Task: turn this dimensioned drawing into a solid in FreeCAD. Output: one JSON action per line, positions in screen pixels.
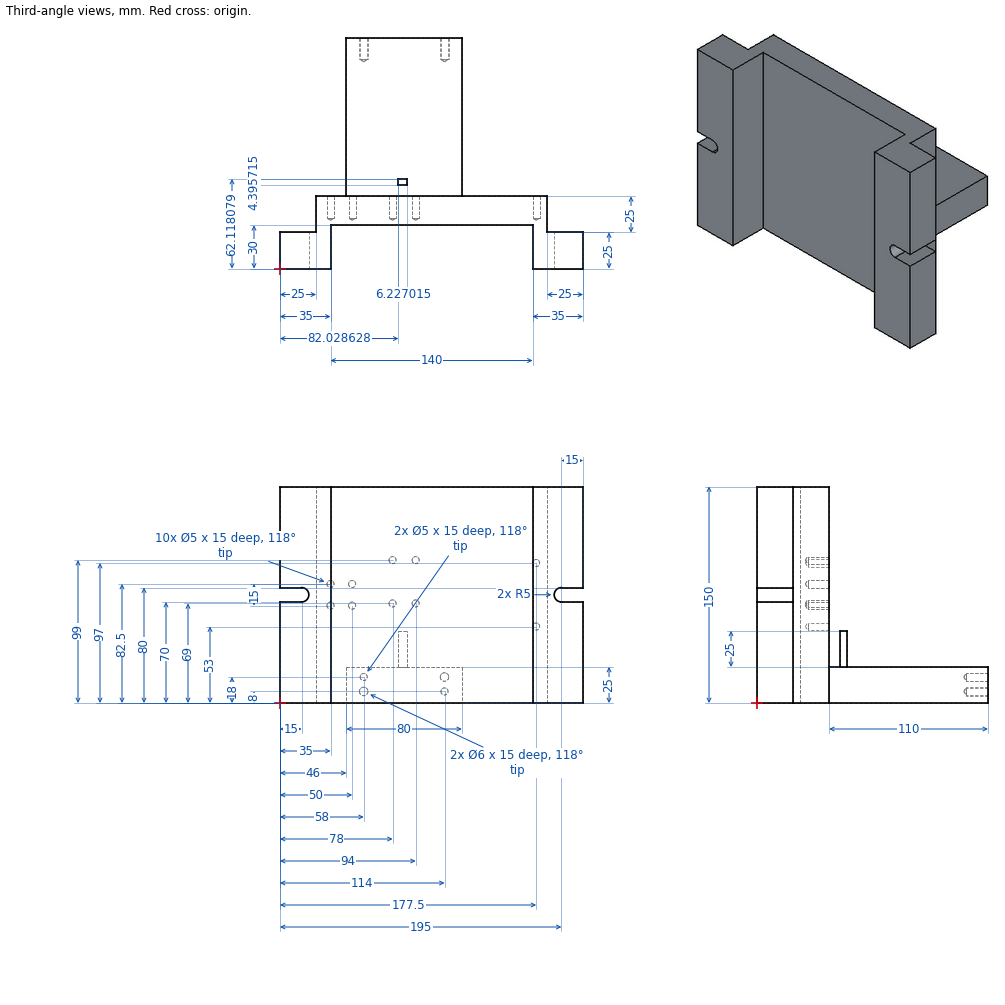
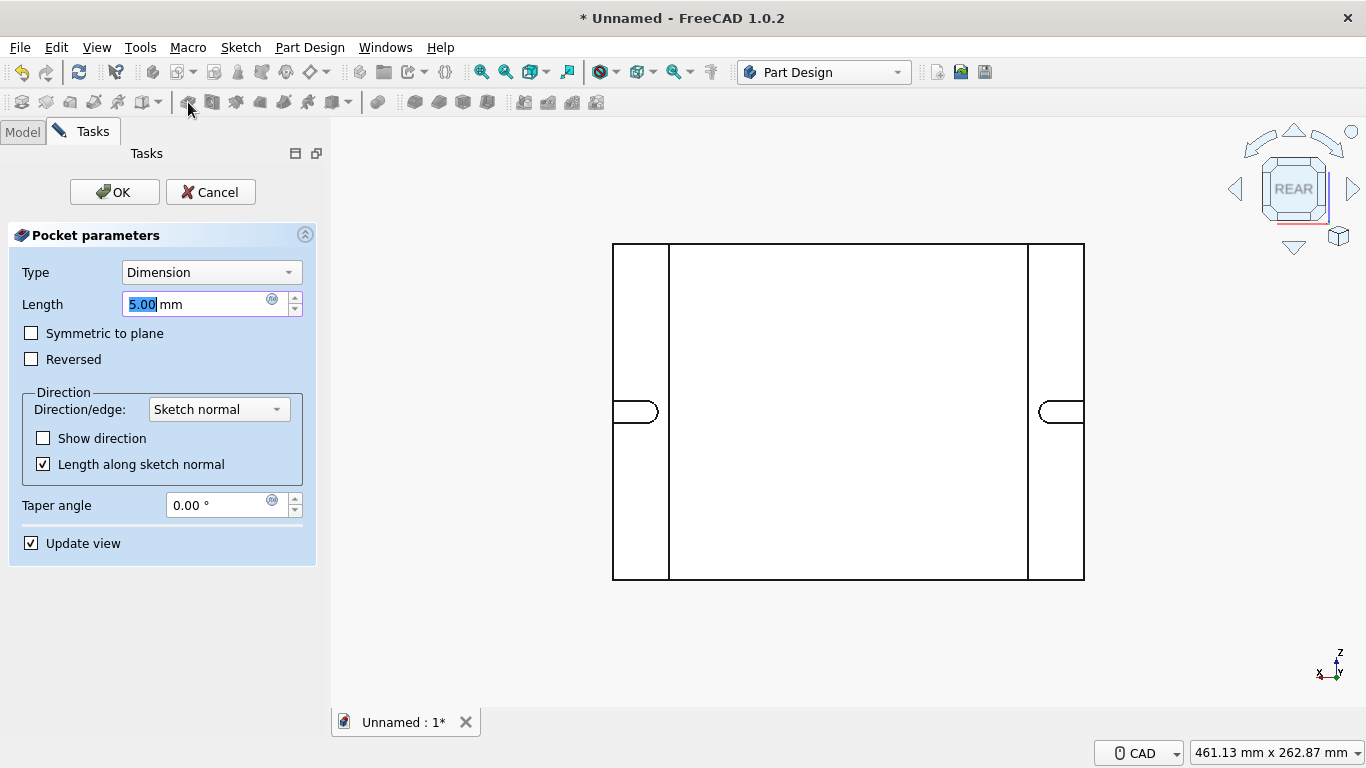
{"action": "left_click", "coordinate": [212, 272]}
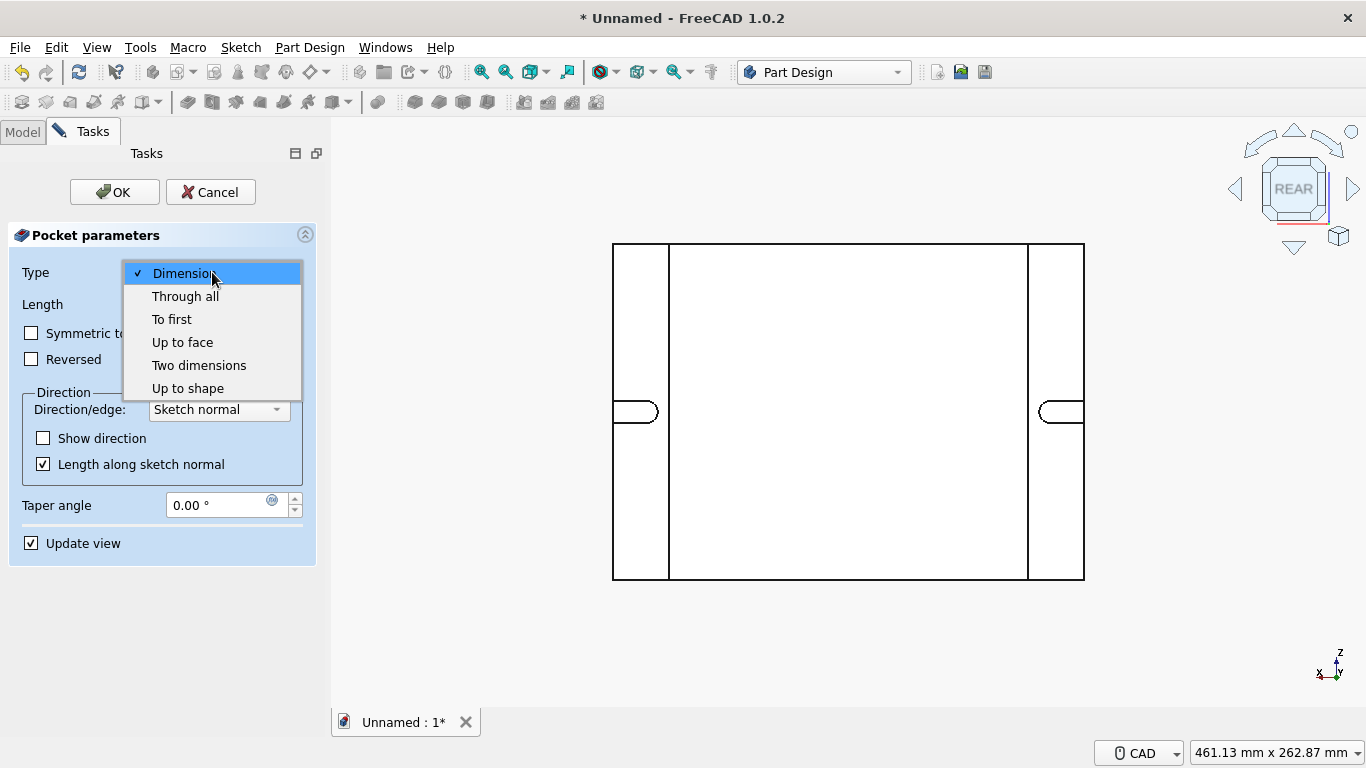
{"action": "left_click", "coordinate": [212, 296]}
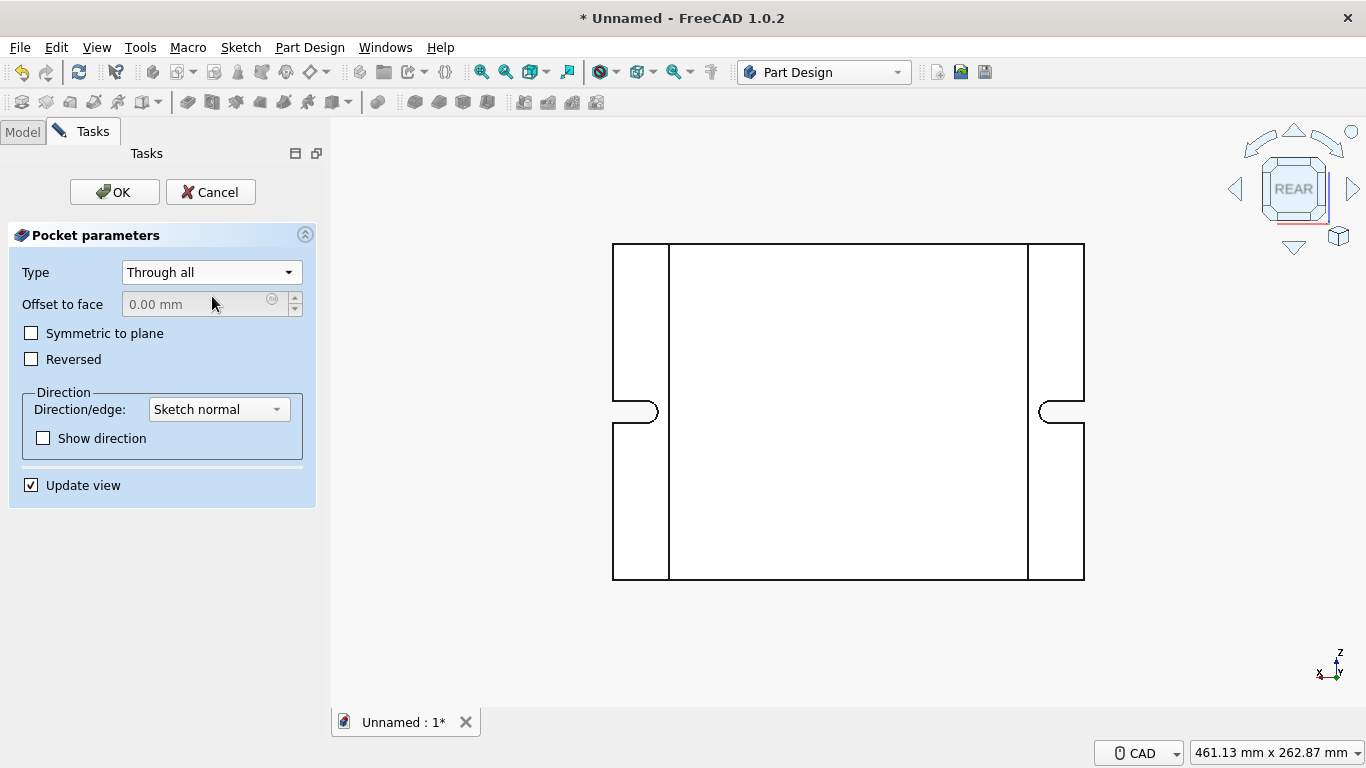
{"action": "left_click", "coordinate": [115, 192]}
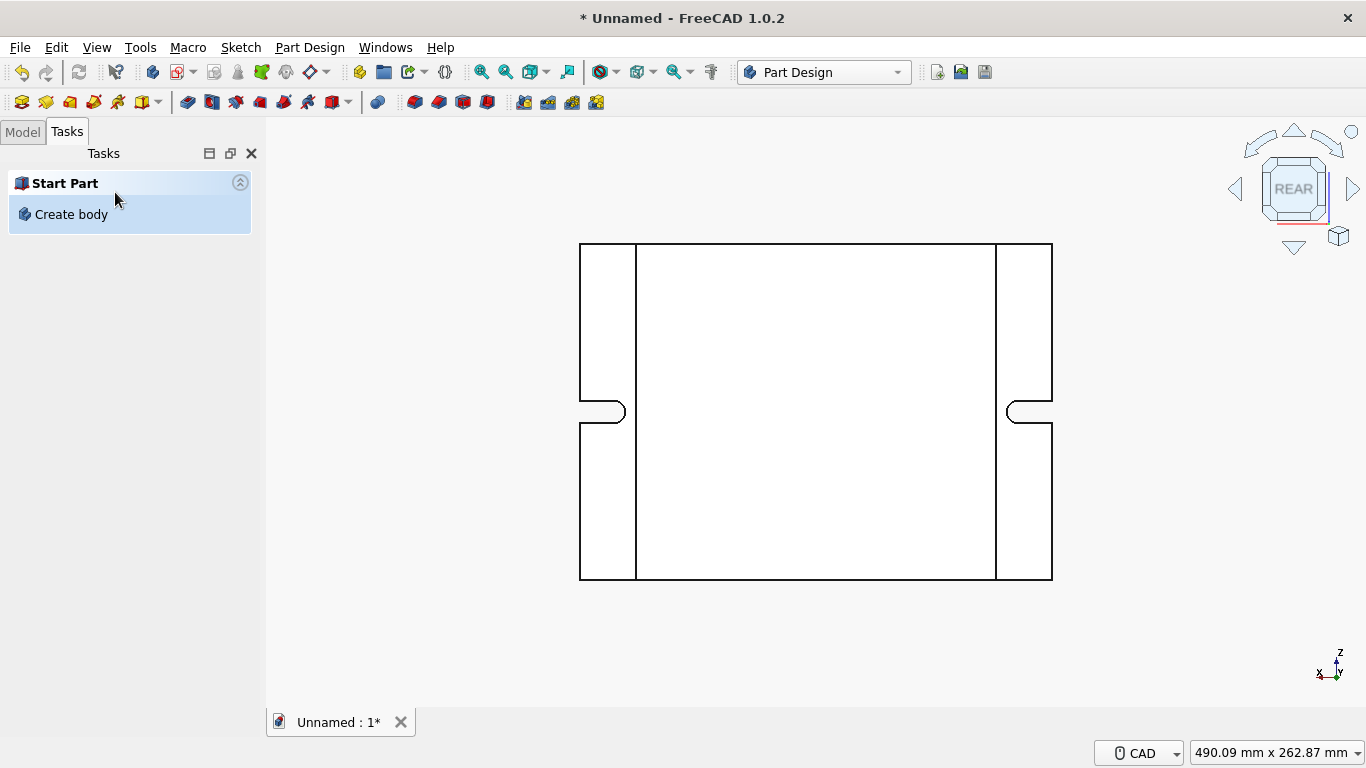
{"action": "left_click", "coordinate": [816, 411]}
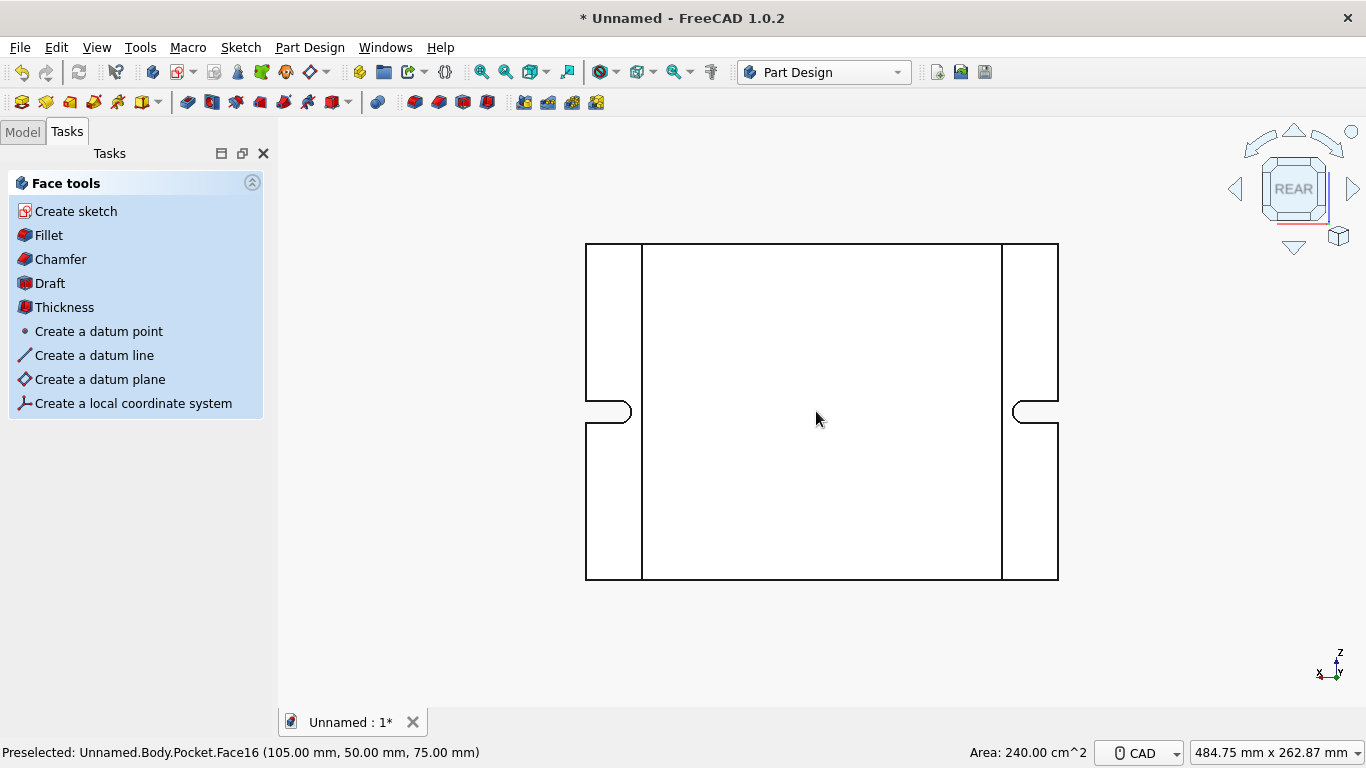
{"action": "left_click", "coordinate": [178, 72]}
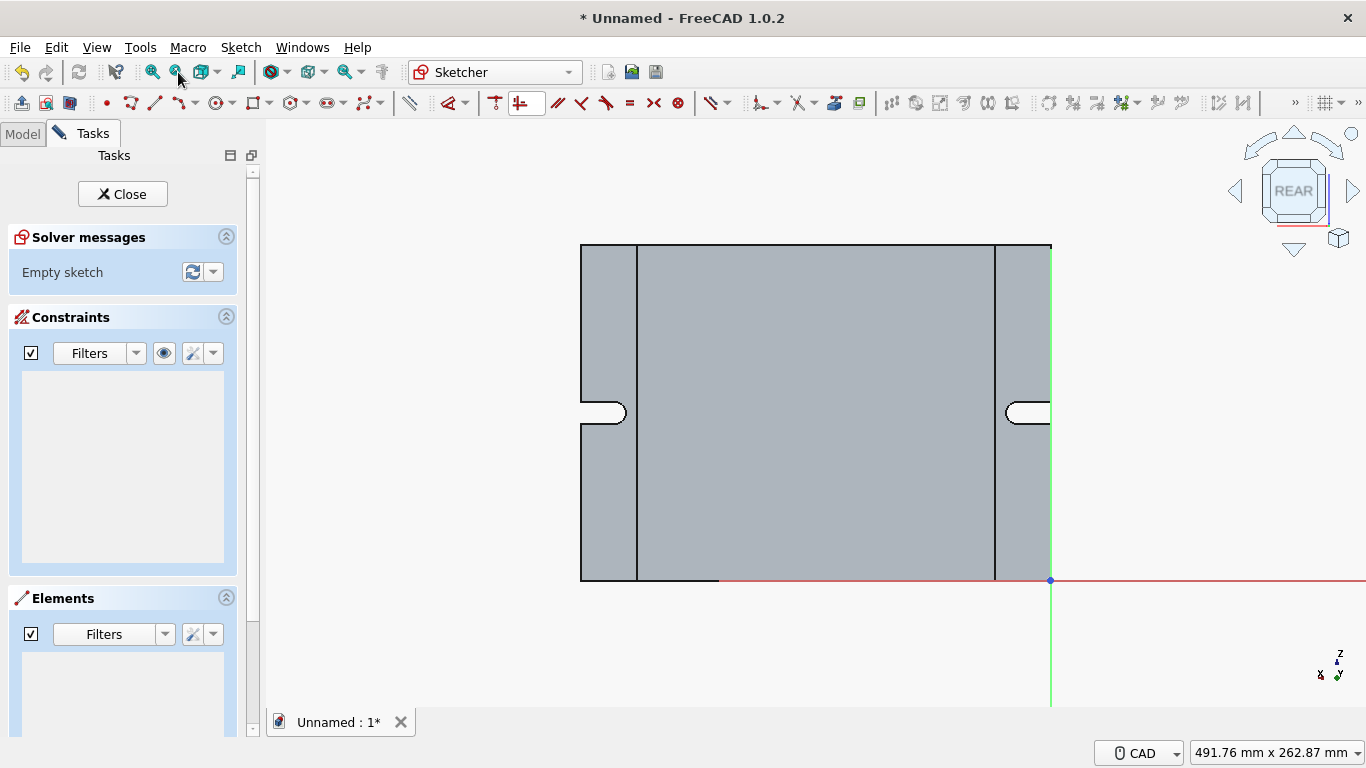
{"action": "scroll", "coordinate": [1057, 578], "scroll_direction": "up", "scroll_amount": 2}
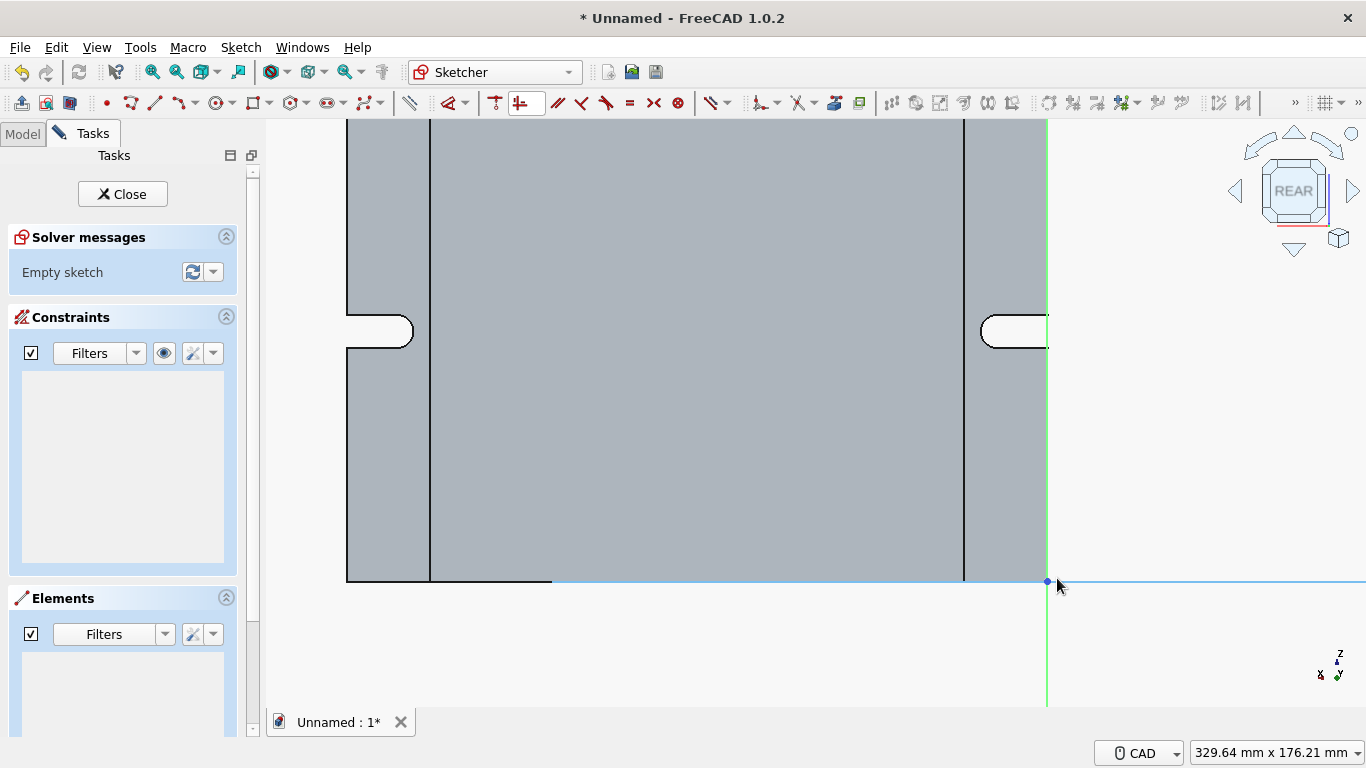
{"action": "left_click", "coordinate": [216, 104]}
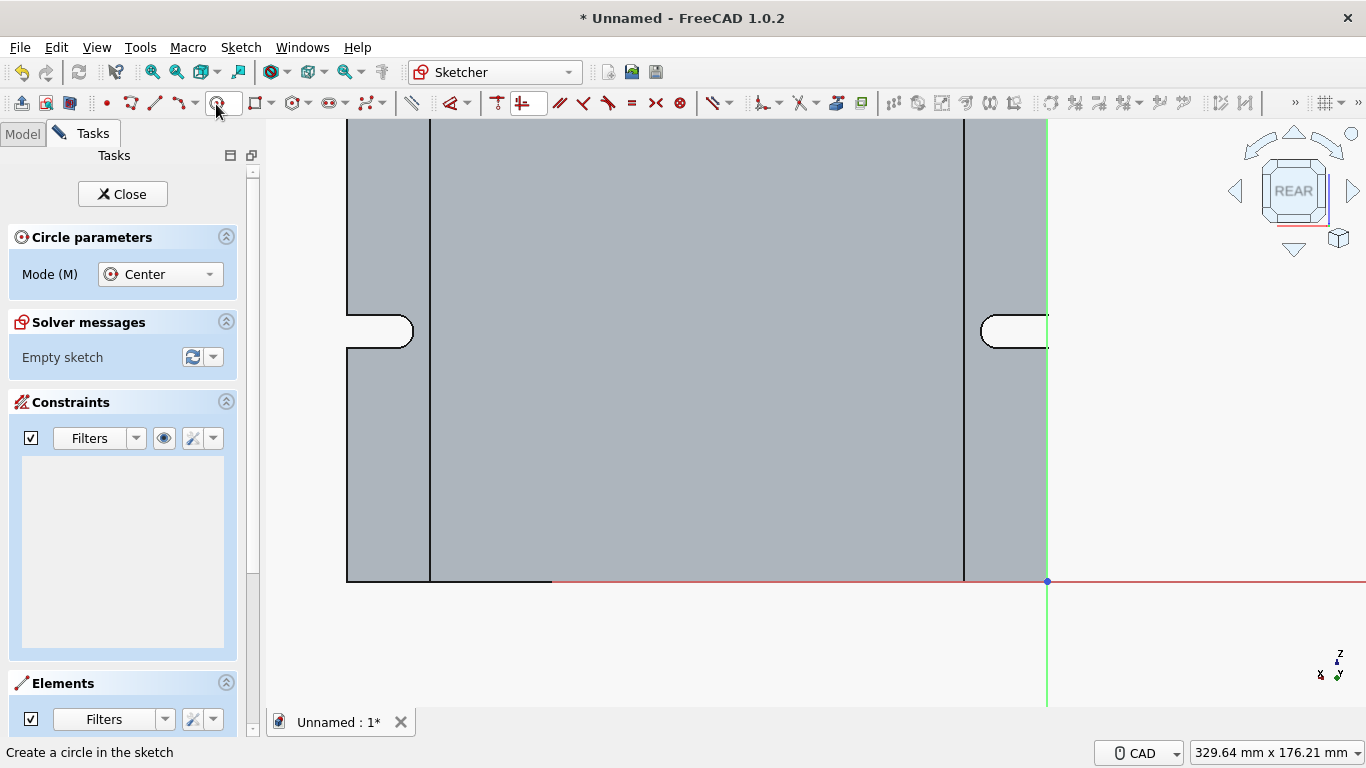
{"action": "scroll", "coordinate": [931, 306], "scroll_direction": "up", "scroll_amount": 6}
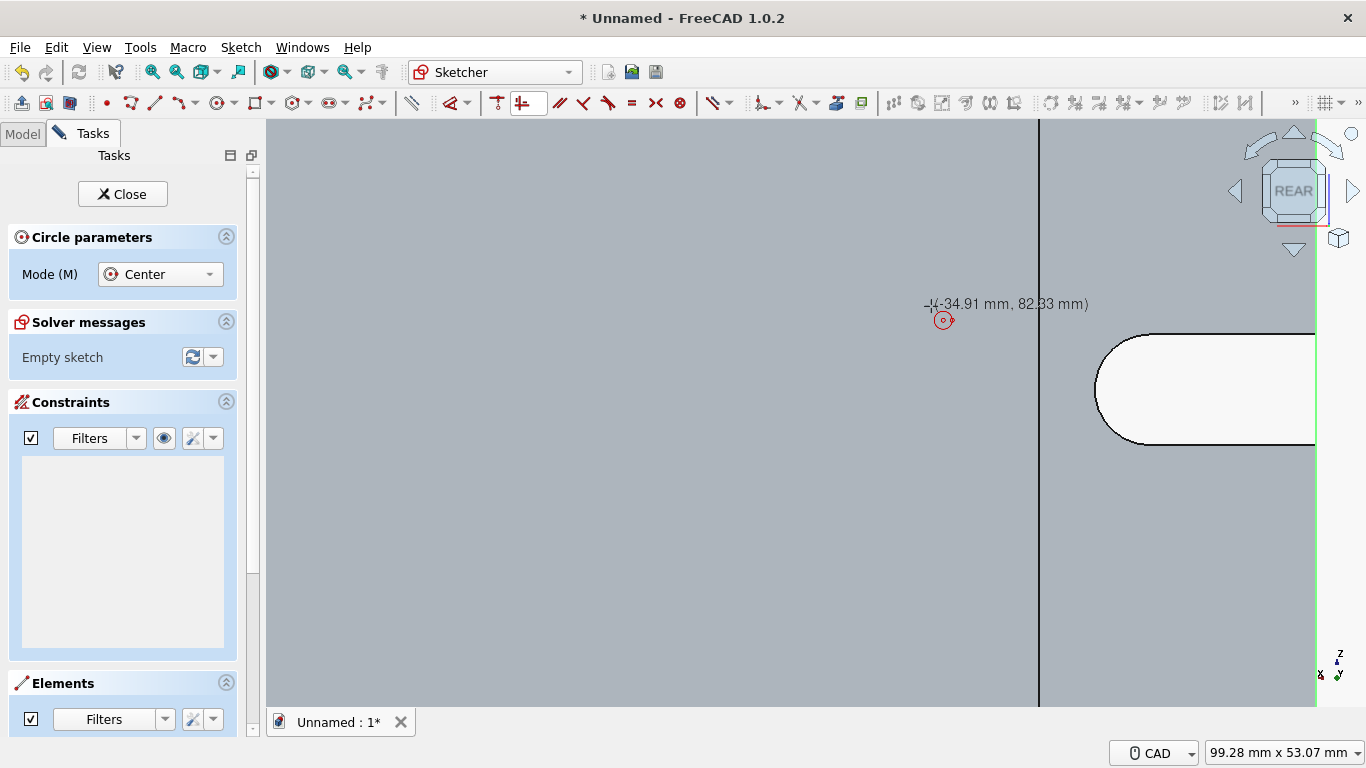
{"action": "left_click", "coordinate": [929, 307]}
{"action": "mouse_move", "coordinate": [948, 287]}